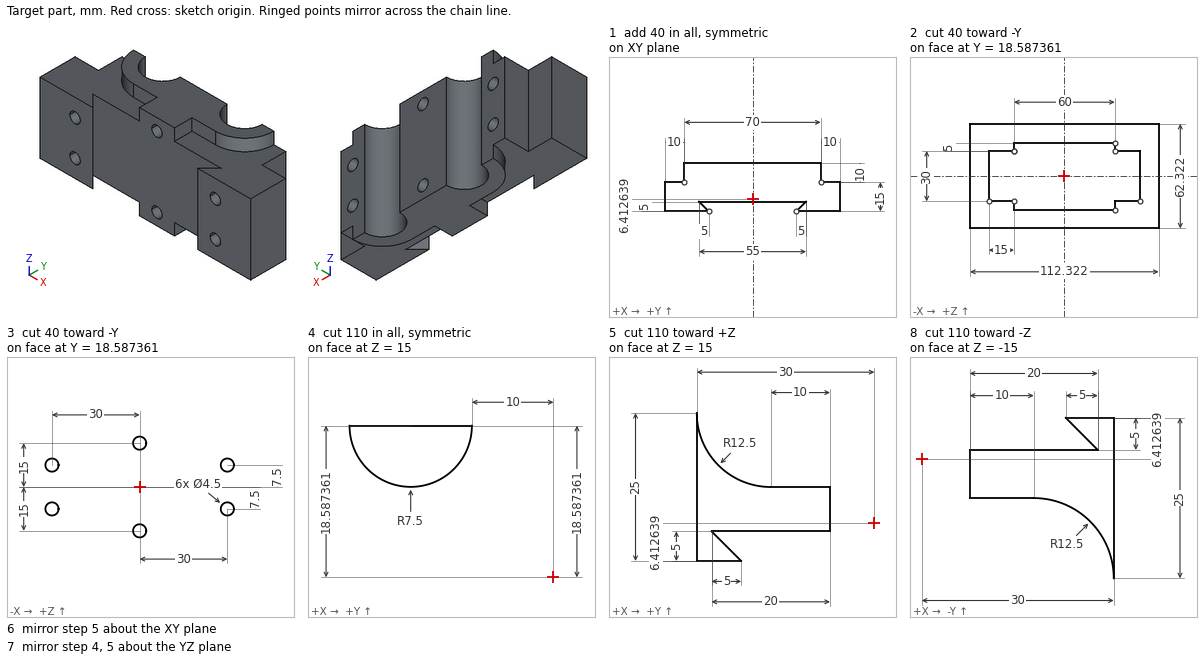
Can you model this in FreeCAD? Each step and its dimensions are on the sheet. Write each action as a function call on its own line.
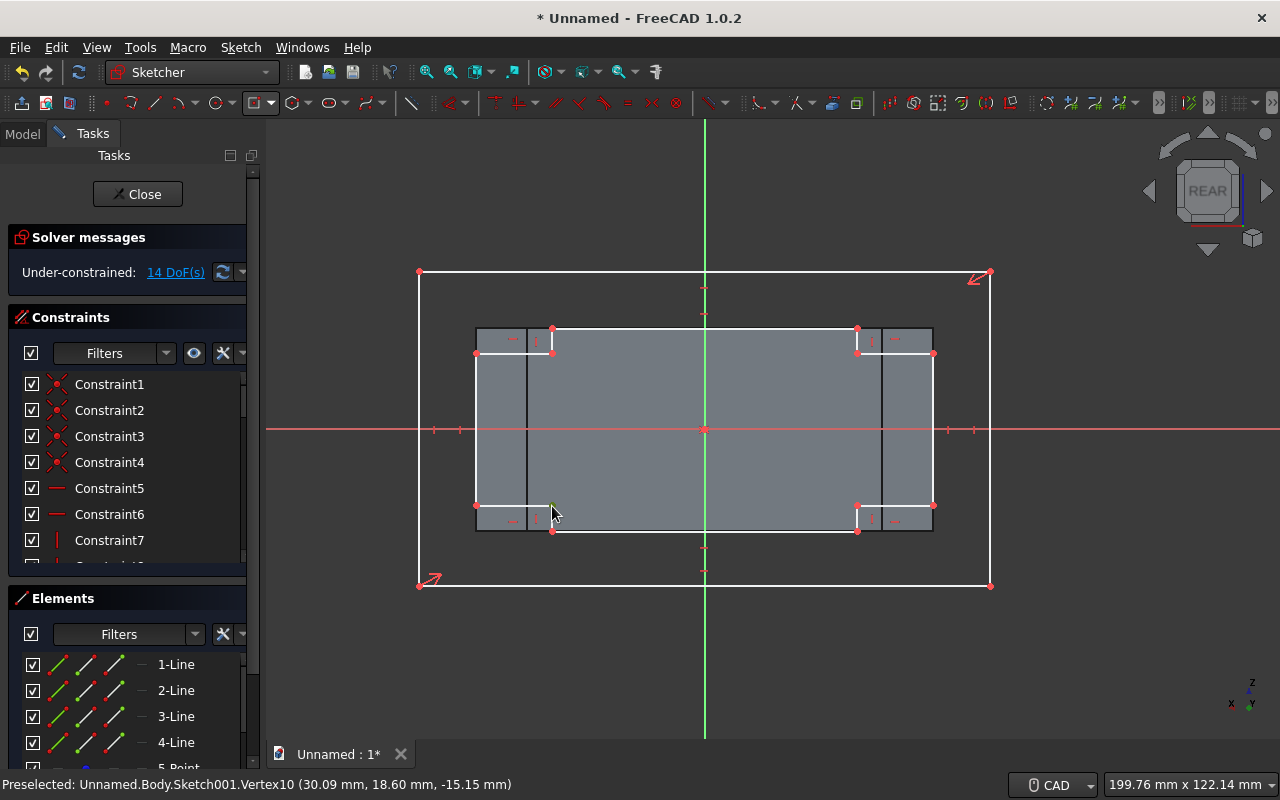
click(552, 354)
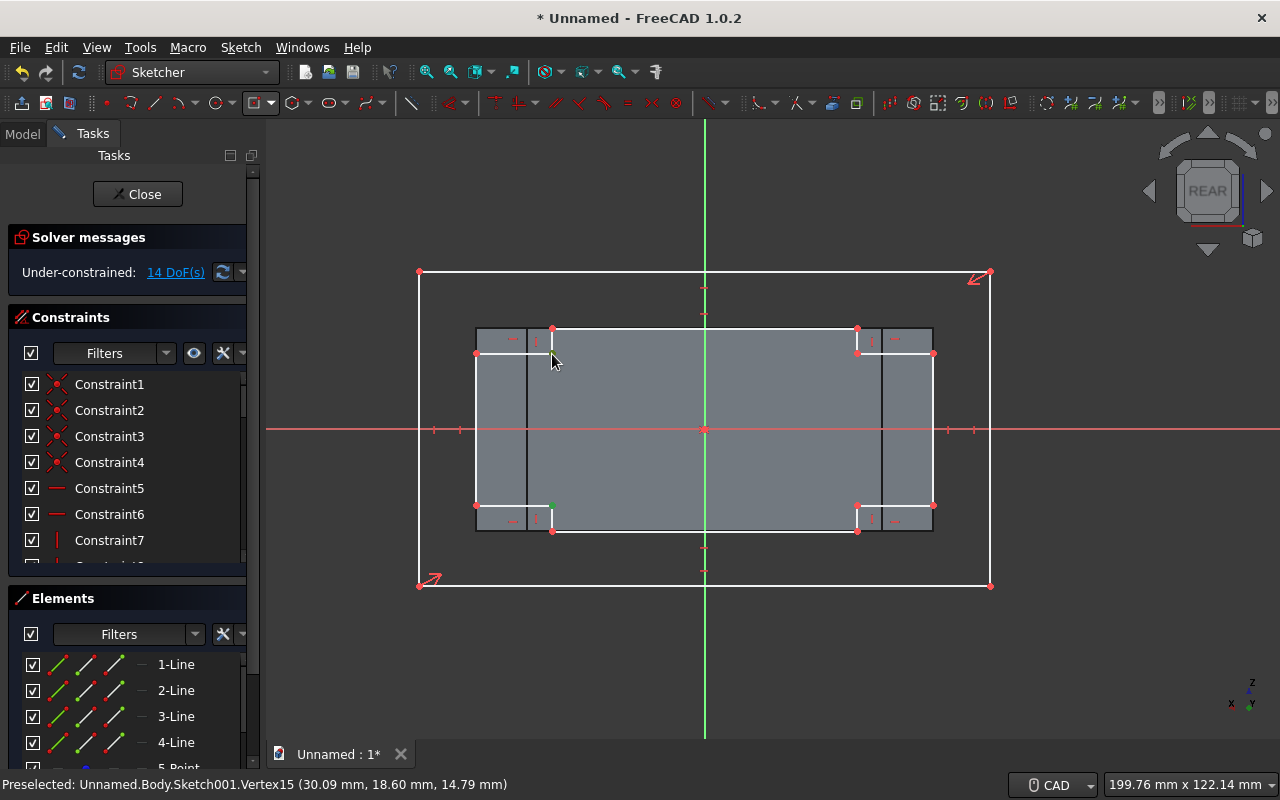
click(353, 429)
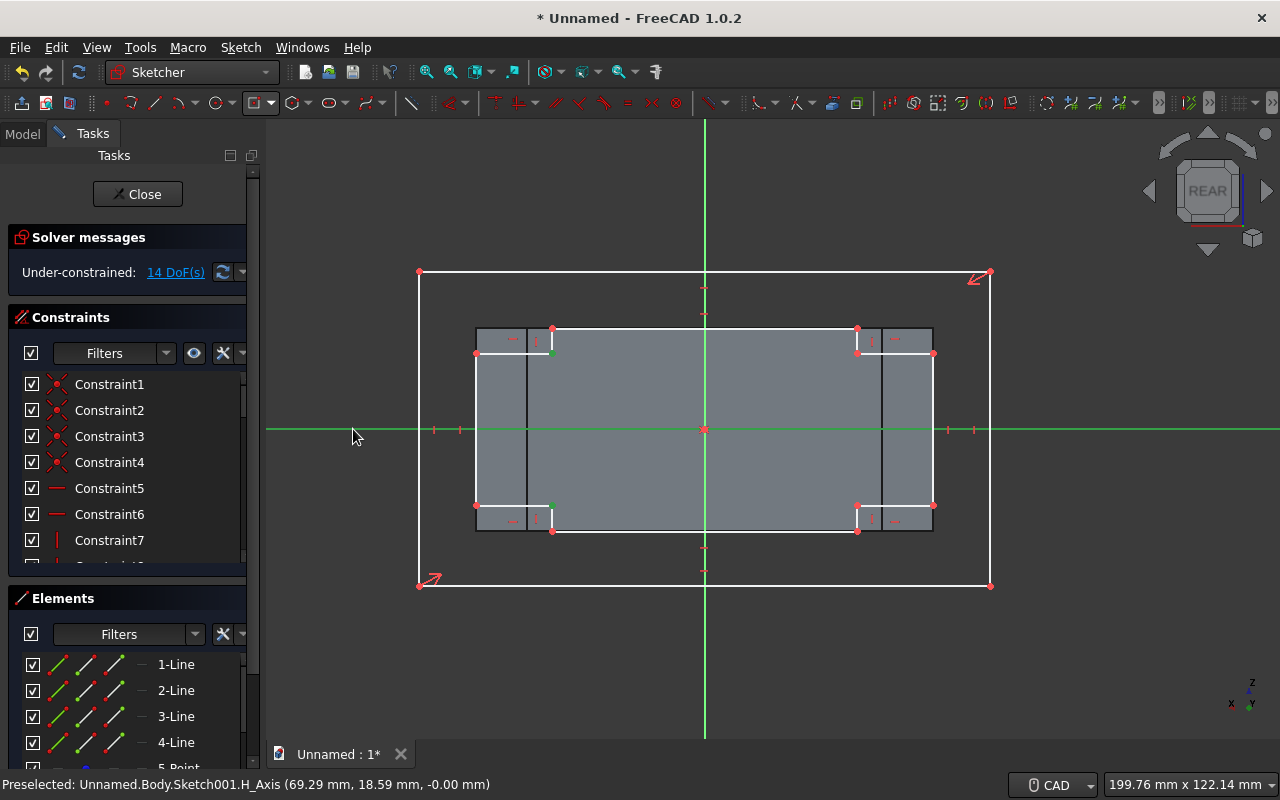
key(s)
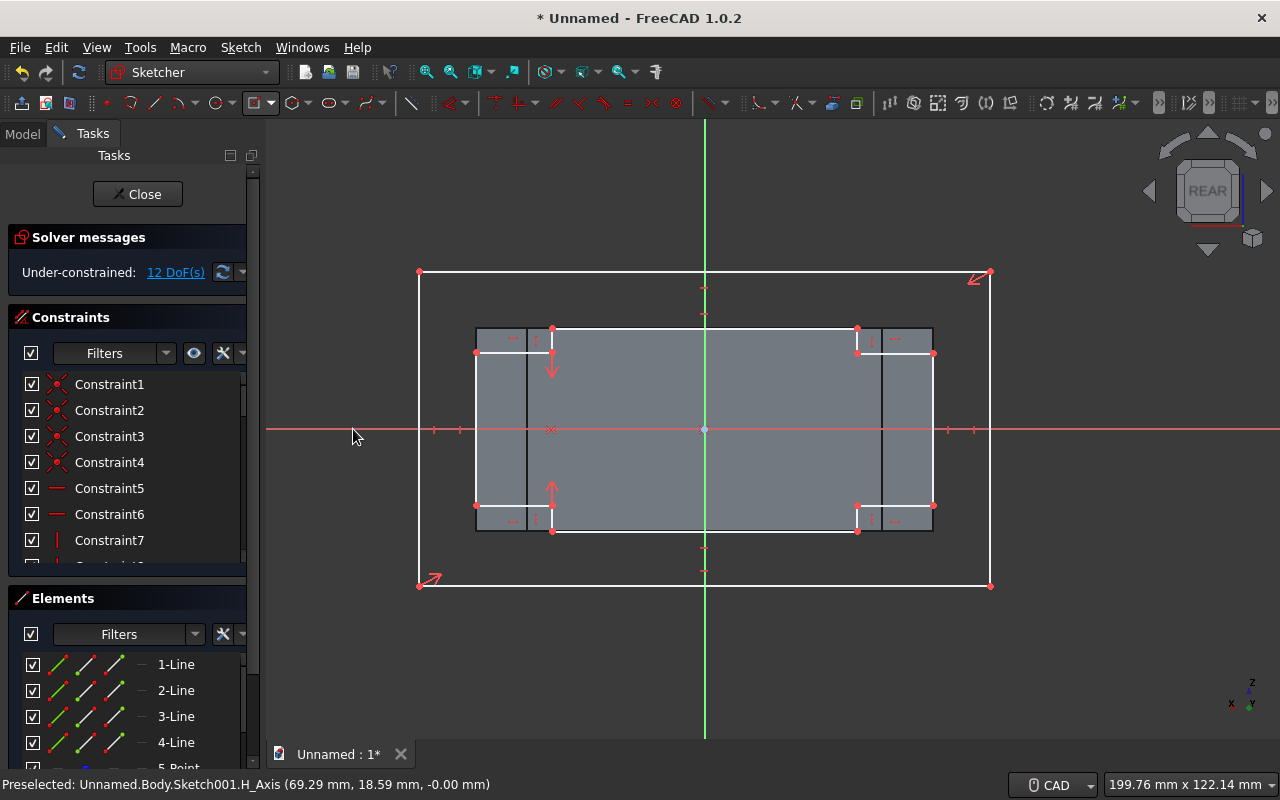
click(552, 353)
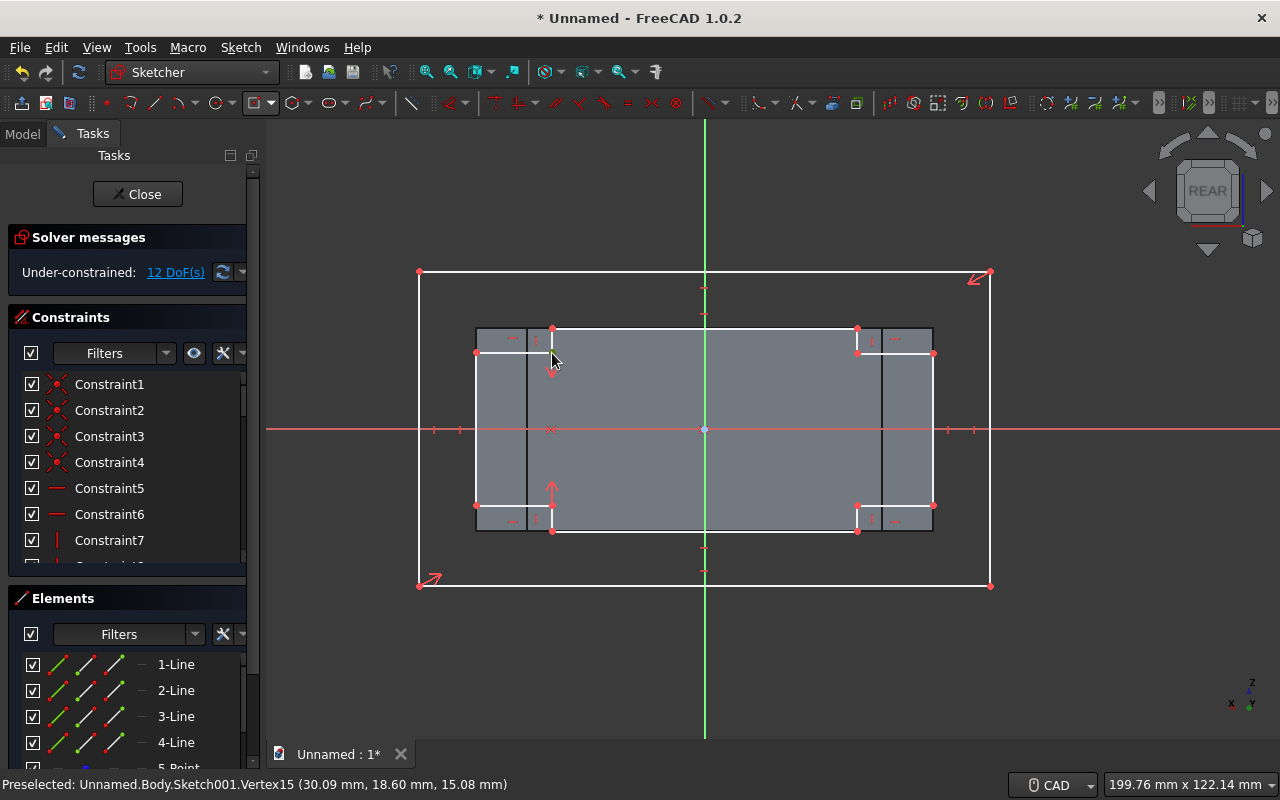
click(857, 354)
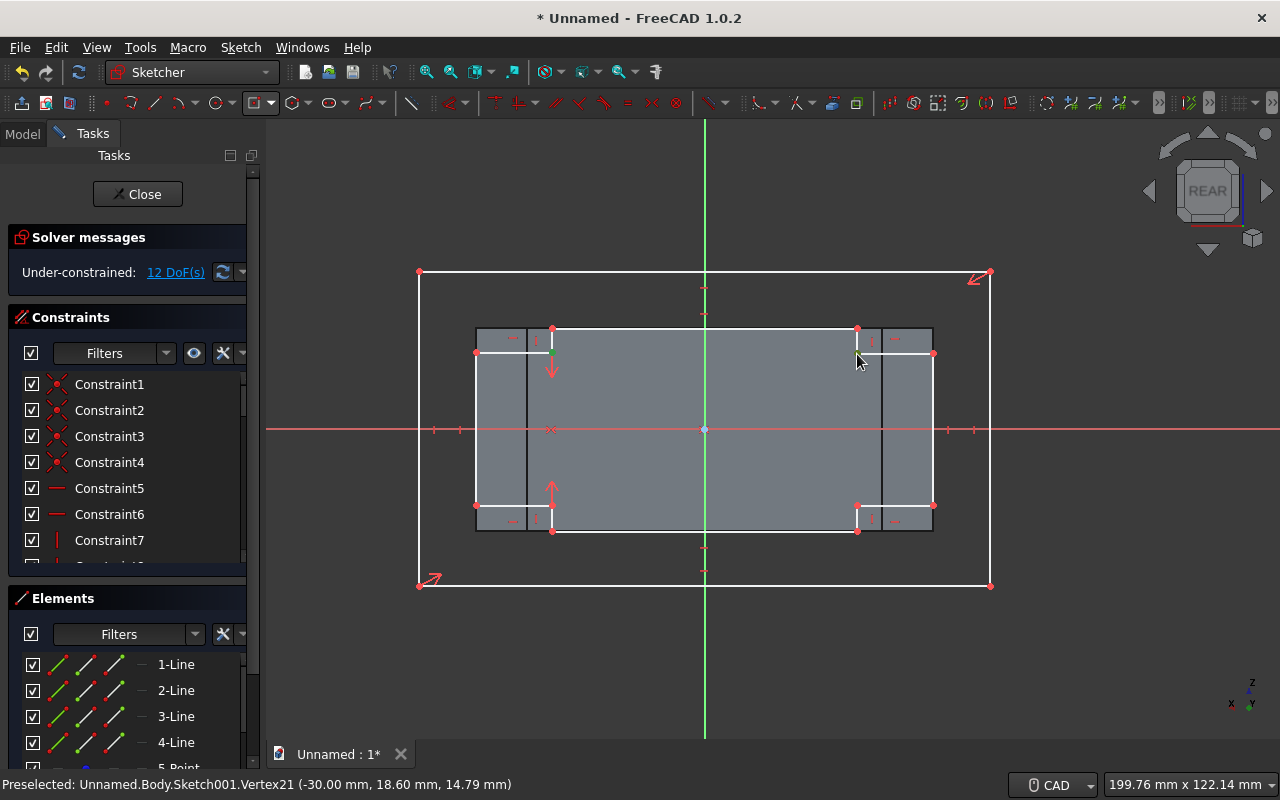
click(705, 671)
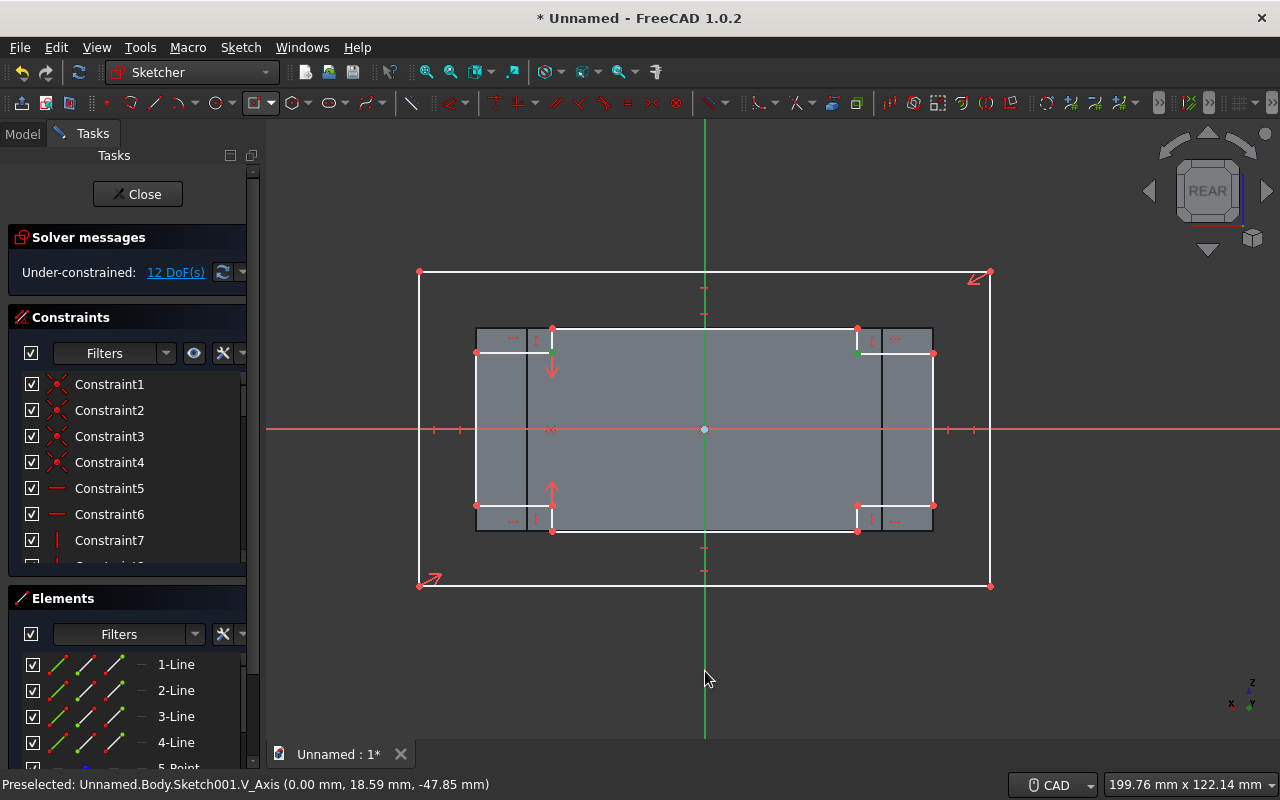
key(s)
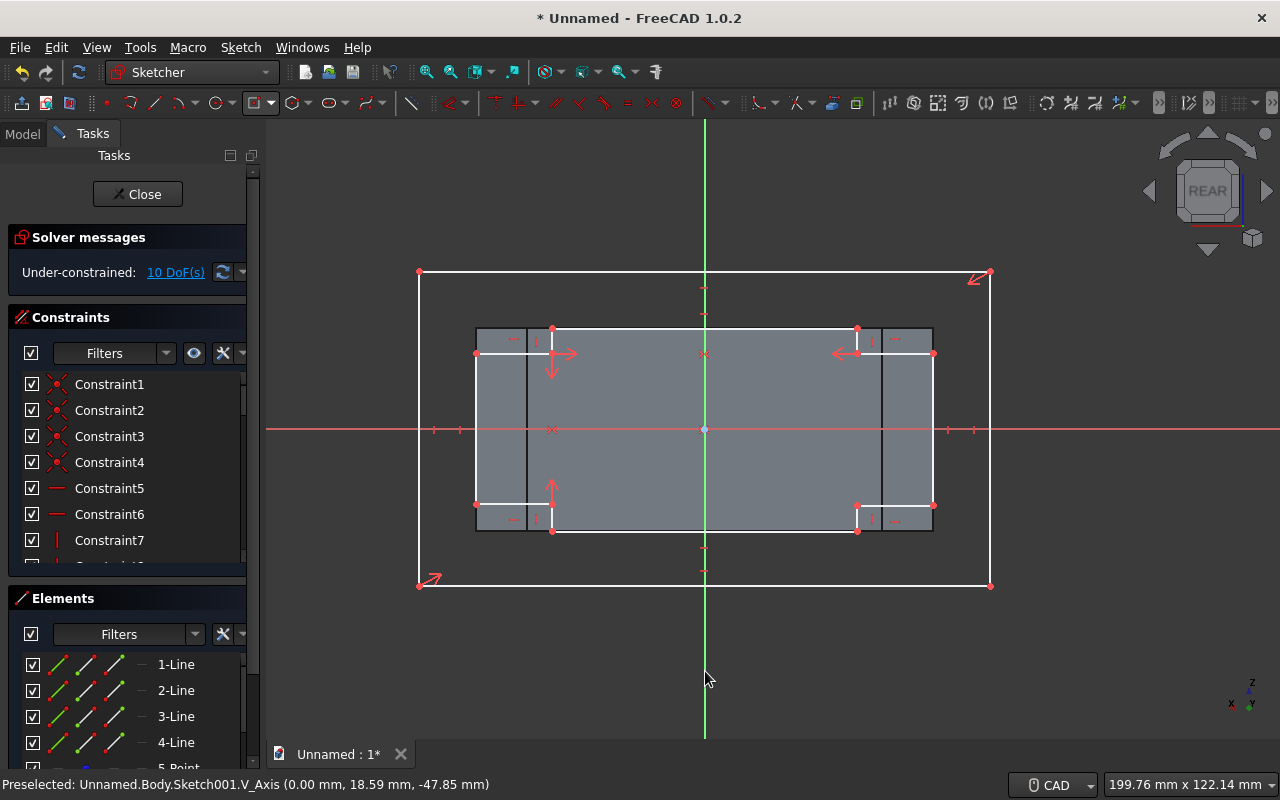
click(476, 504)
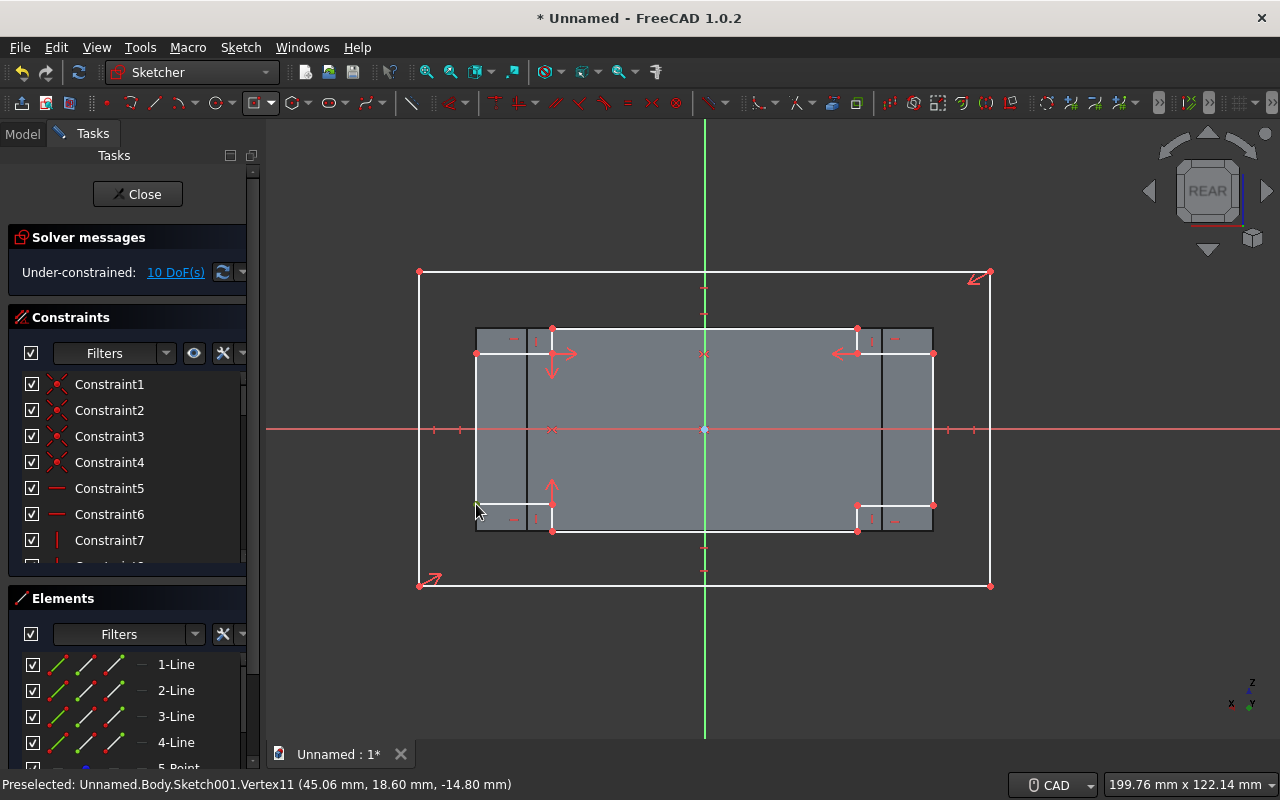
click(933, 506)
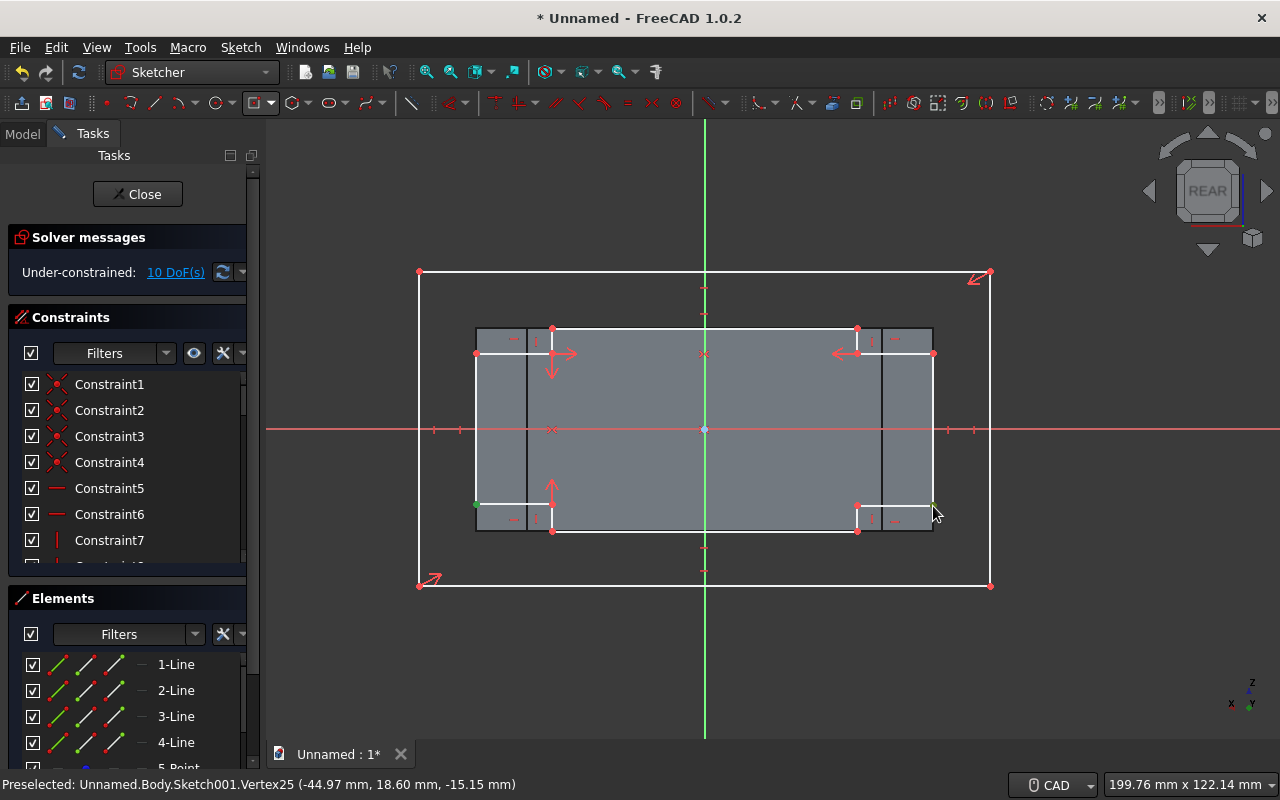
click(705, 671)